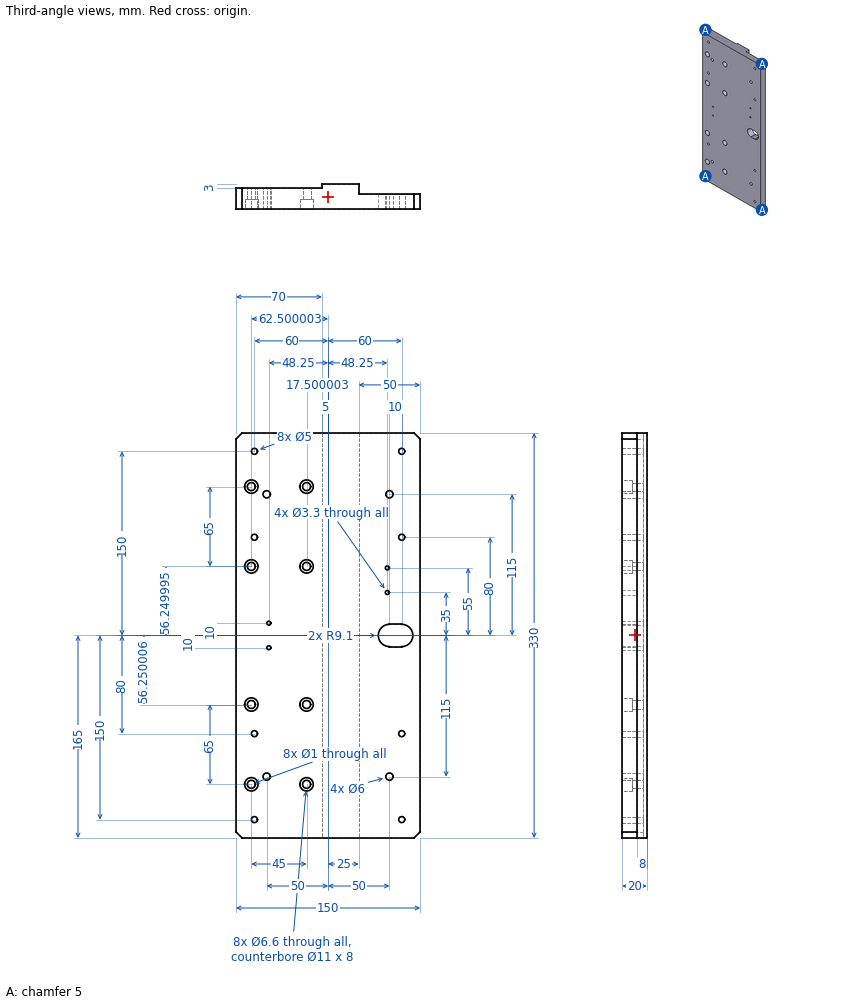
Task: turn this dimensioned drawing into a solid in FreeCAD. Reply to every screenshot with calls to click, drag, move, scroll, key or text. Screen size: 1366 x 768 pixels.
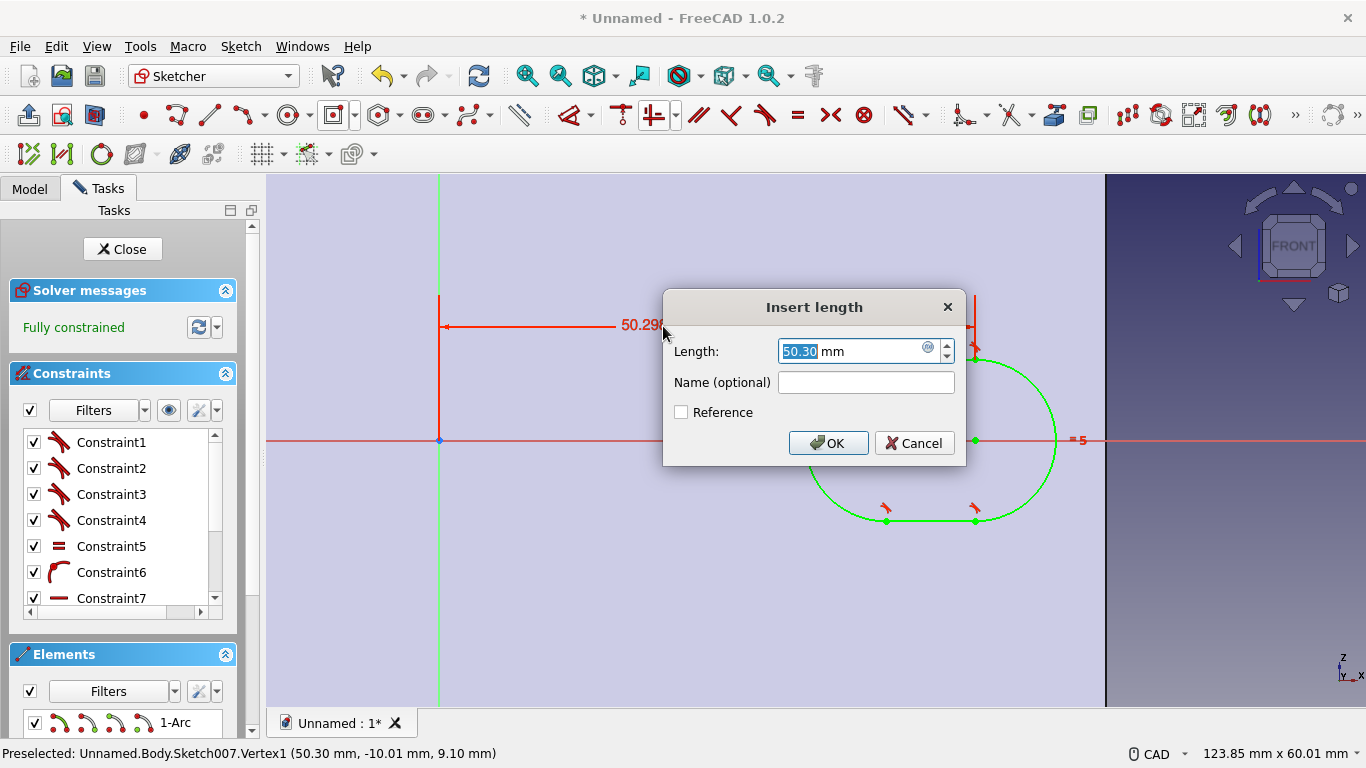
text(50)
key(Return)
key(Escape)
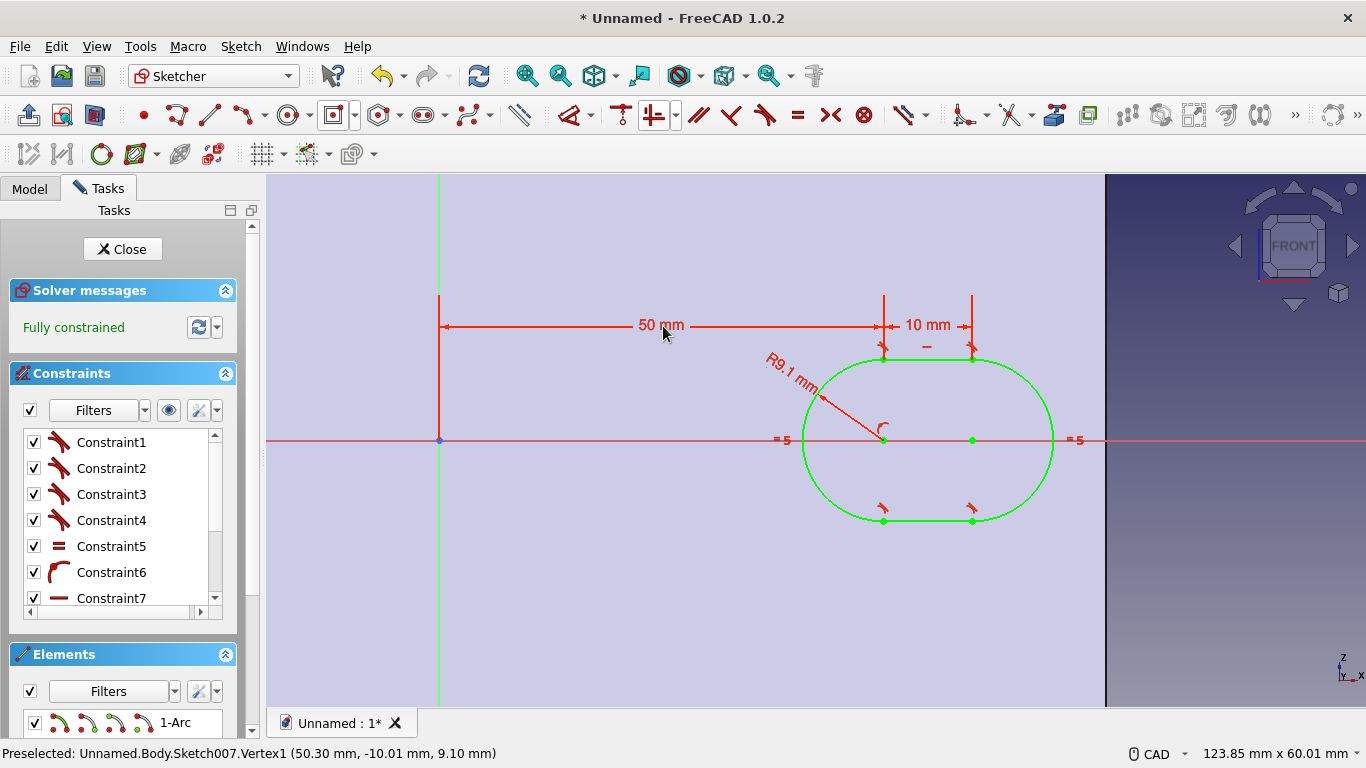
click(123, 249)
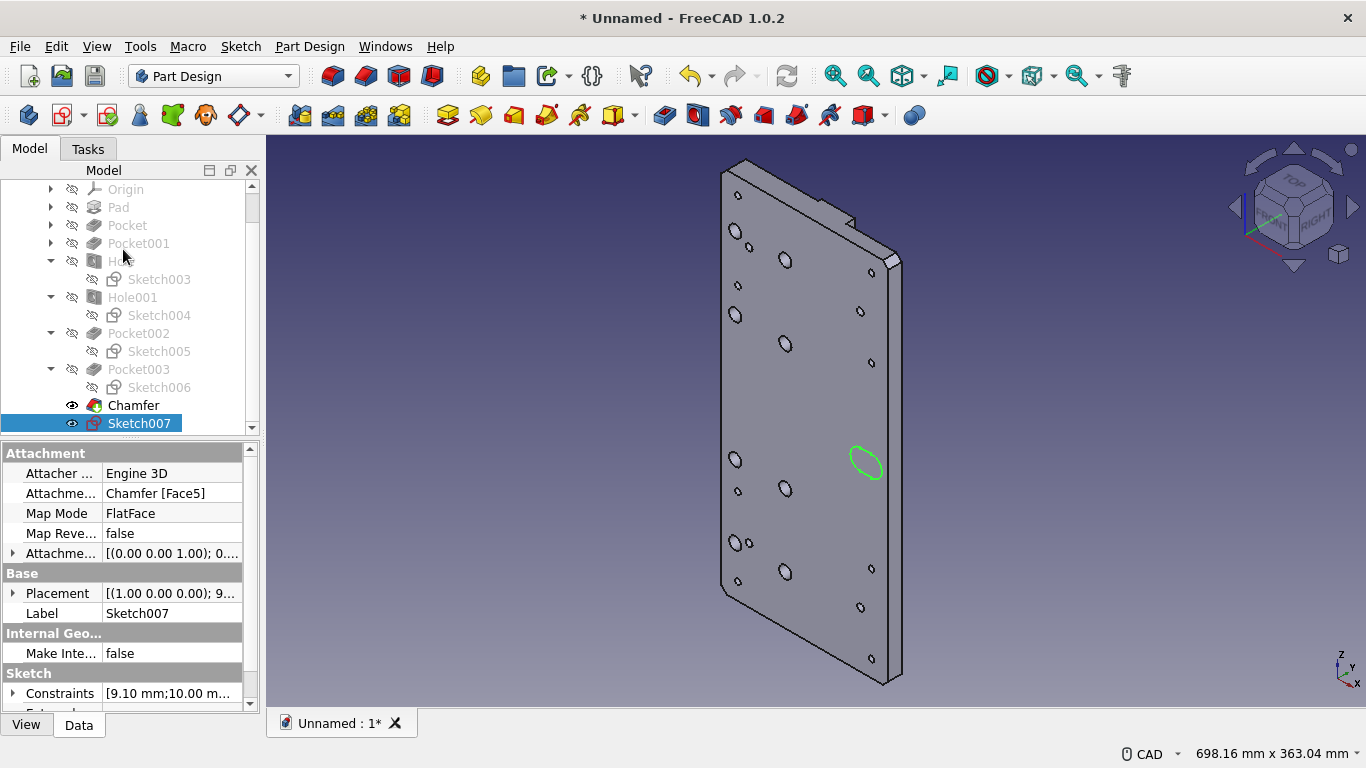
click(665, 116)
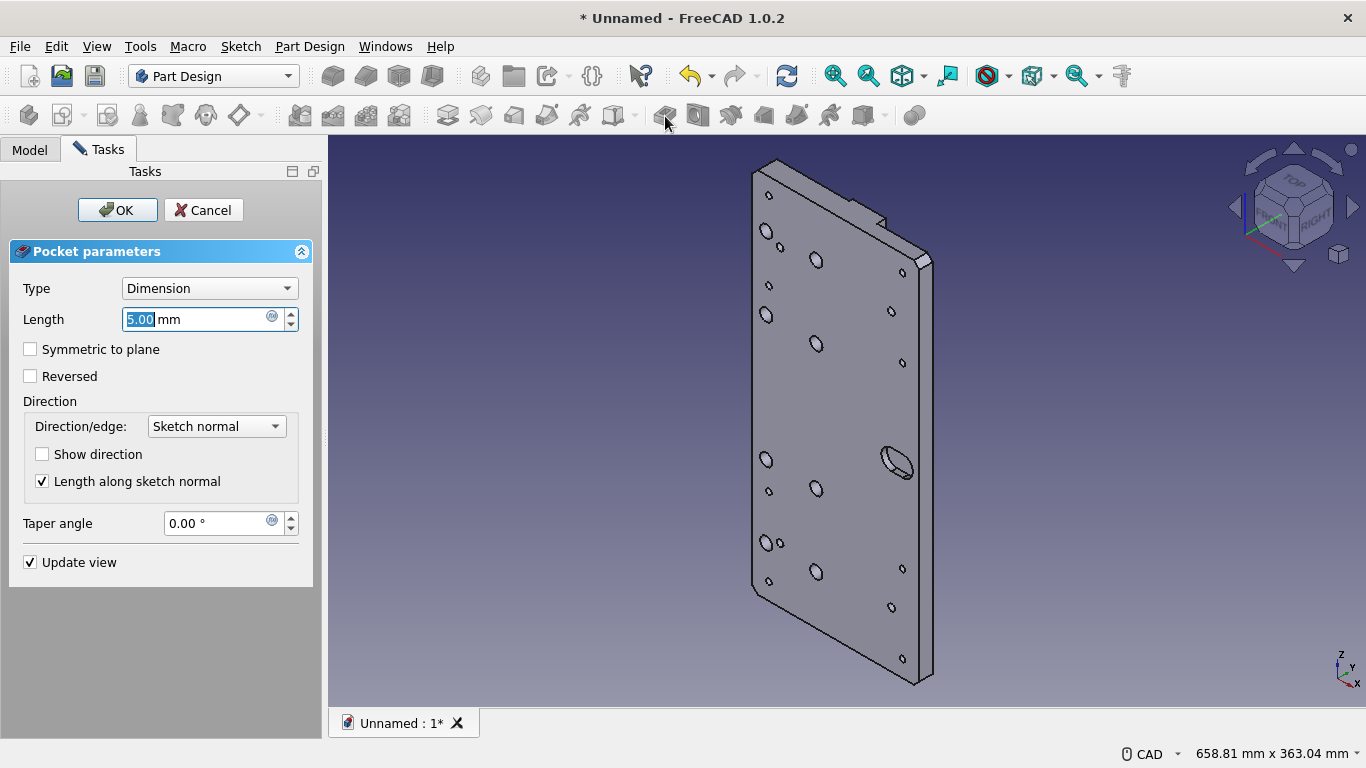
click(210, 288)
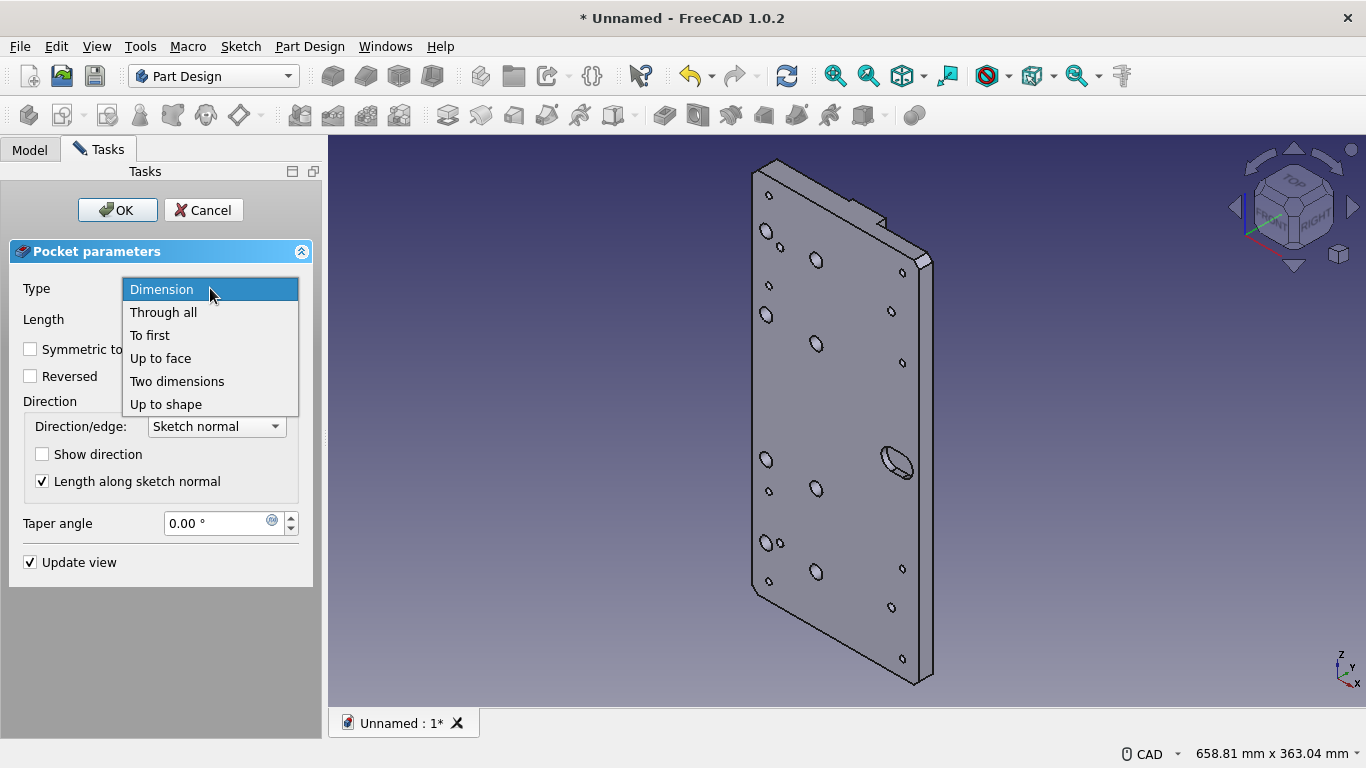
click(208, 312)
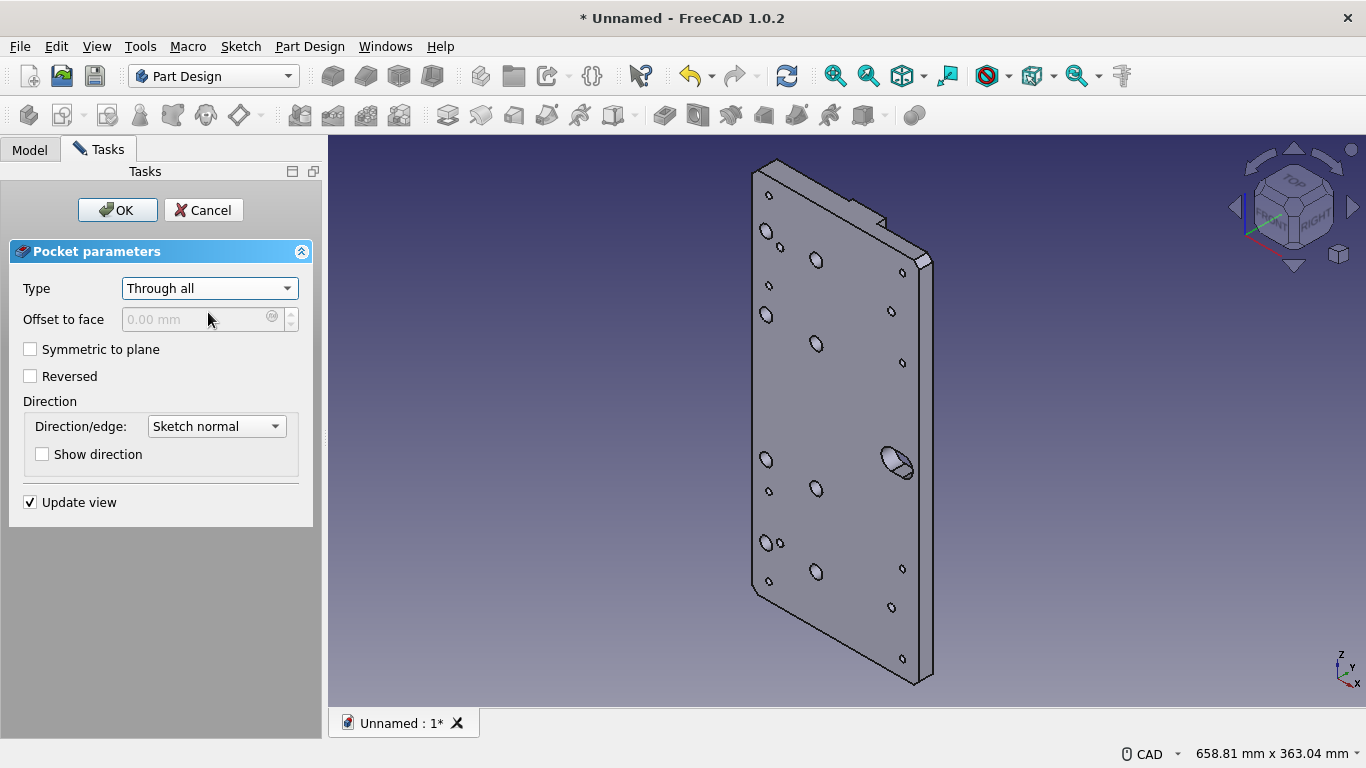
click(118, 210)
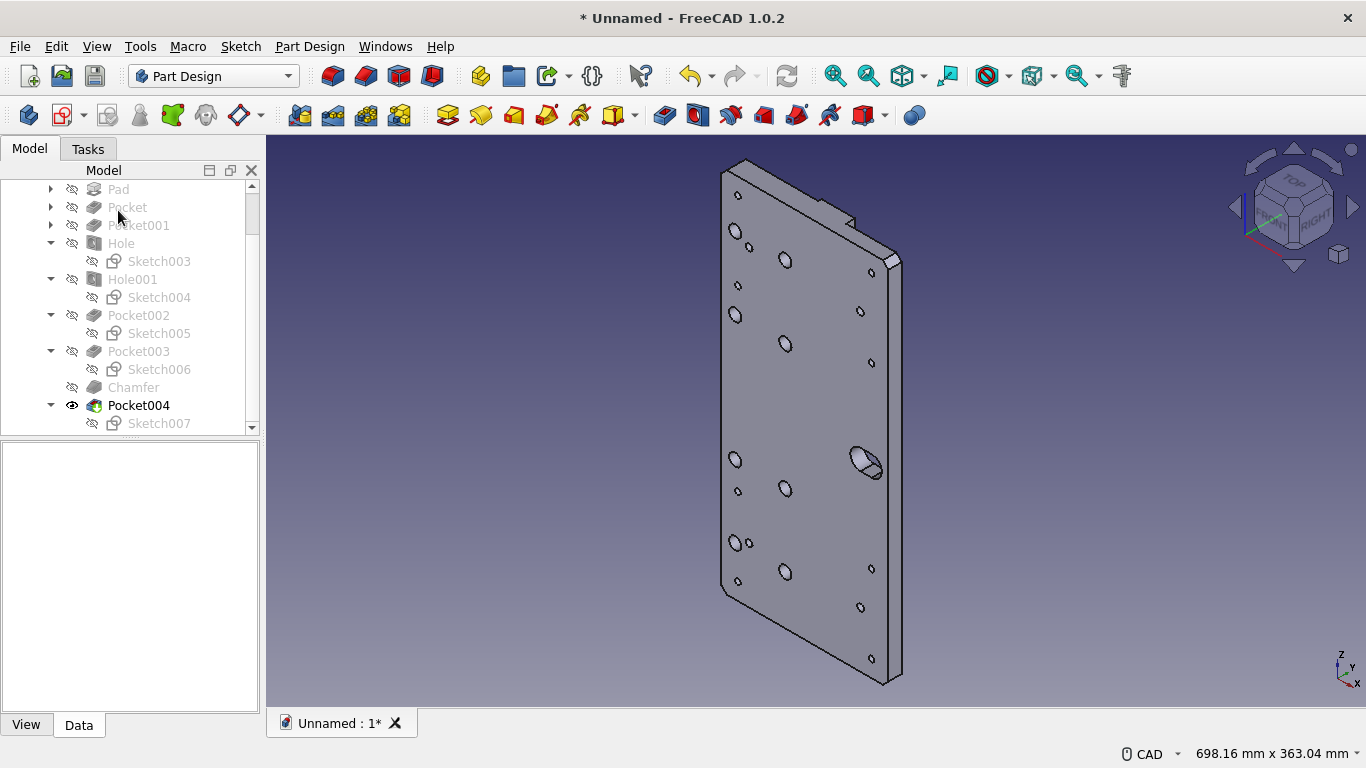
click(781, 413)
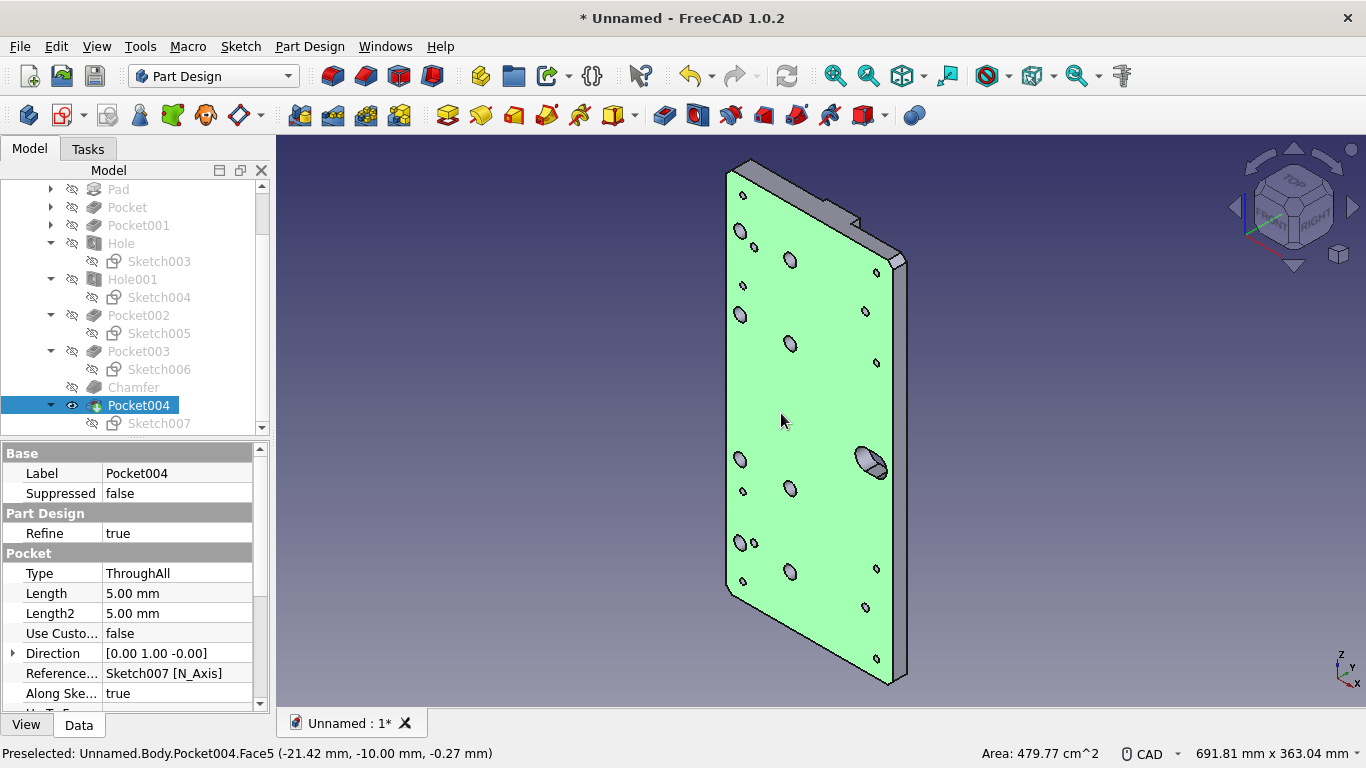
click(62, 116)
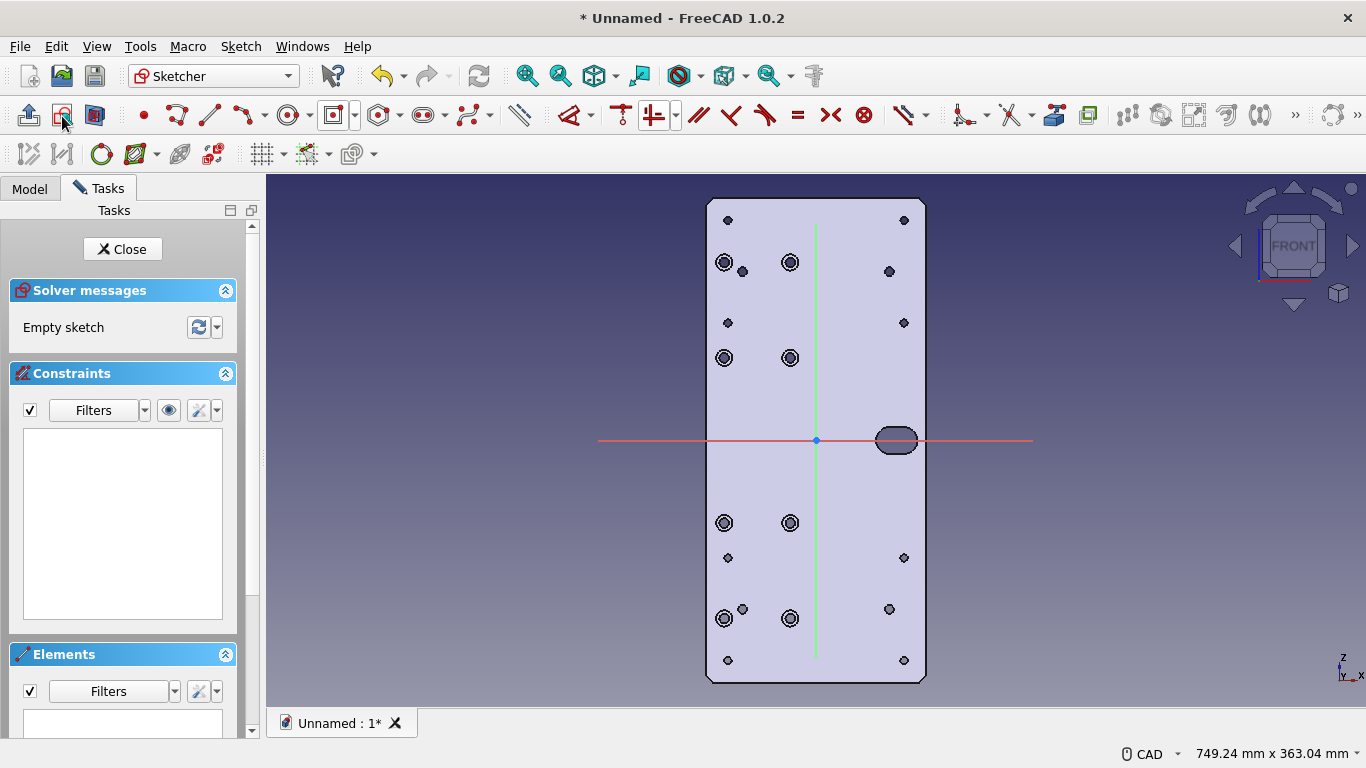
scroll(846, 393, up, 6)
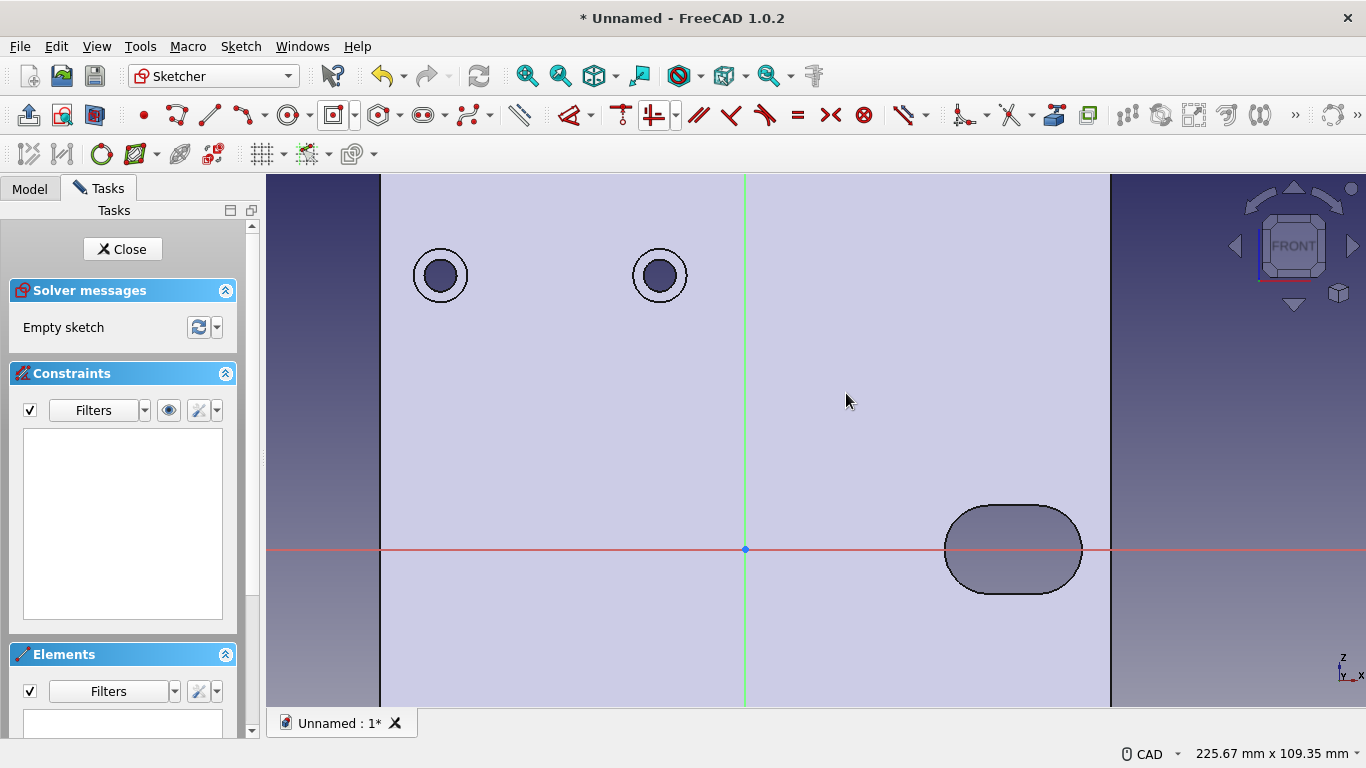
click(288, 116)